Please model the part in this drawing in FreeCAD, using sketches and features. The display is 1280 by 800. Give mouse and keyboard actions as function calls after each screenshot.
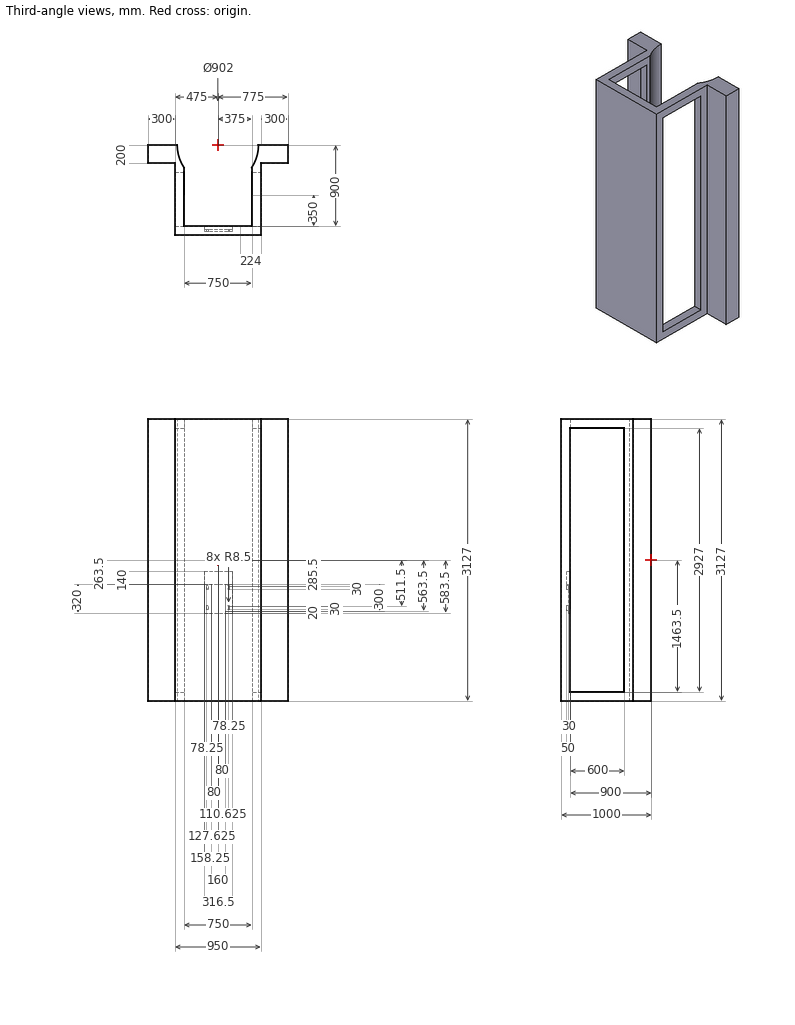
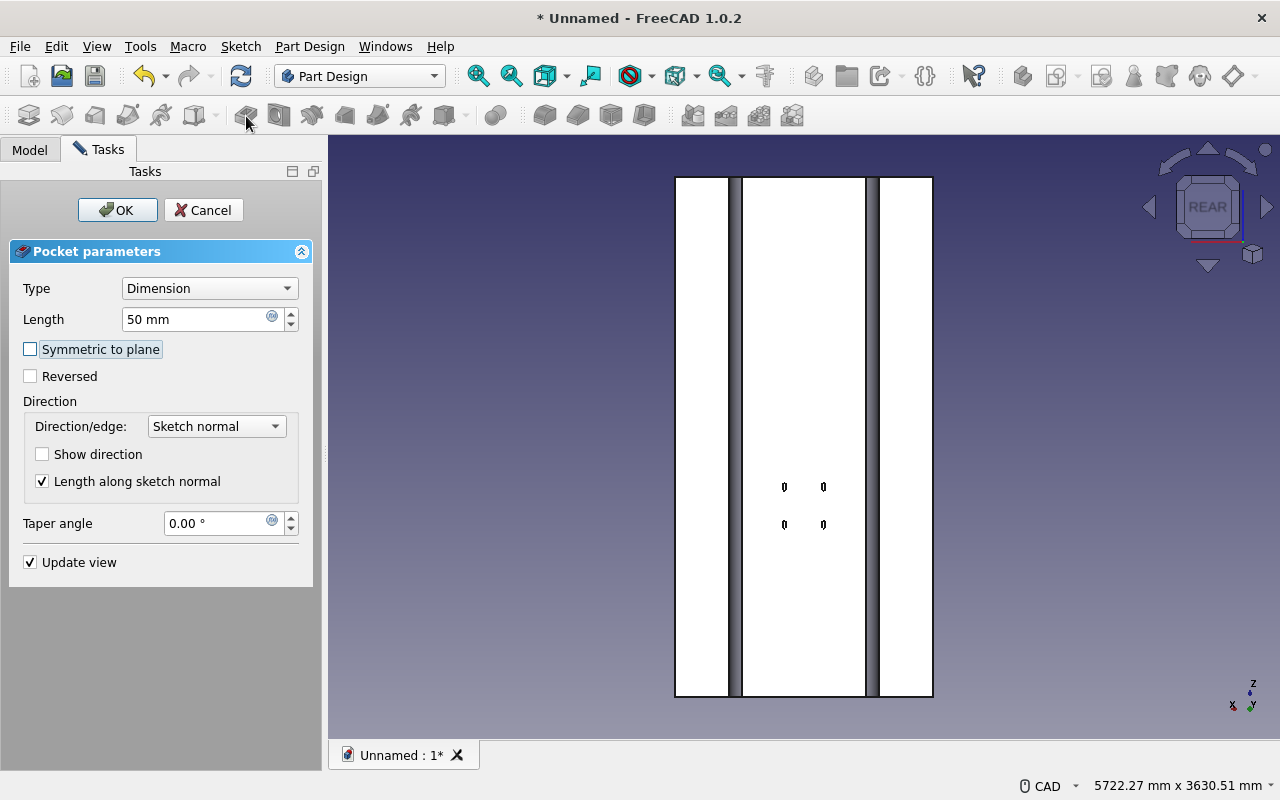
click(118, 210)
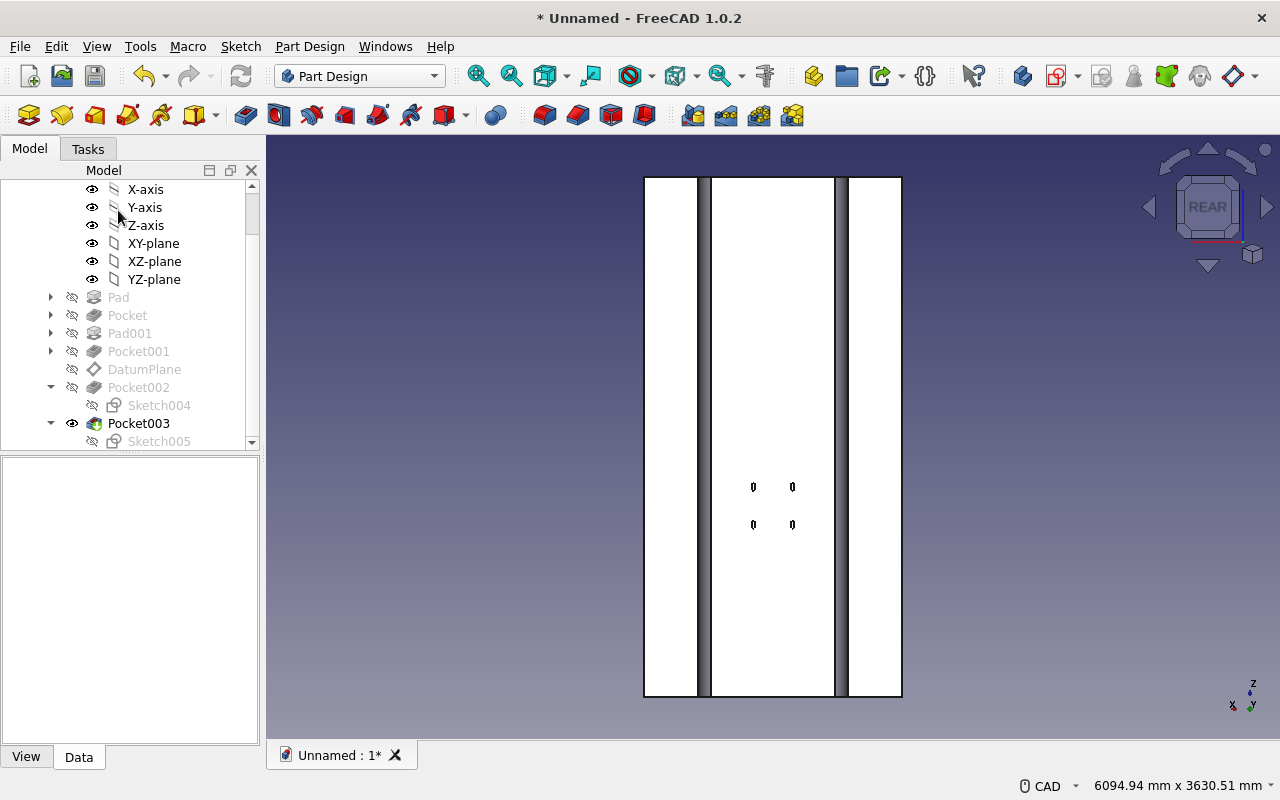
click(773, 287)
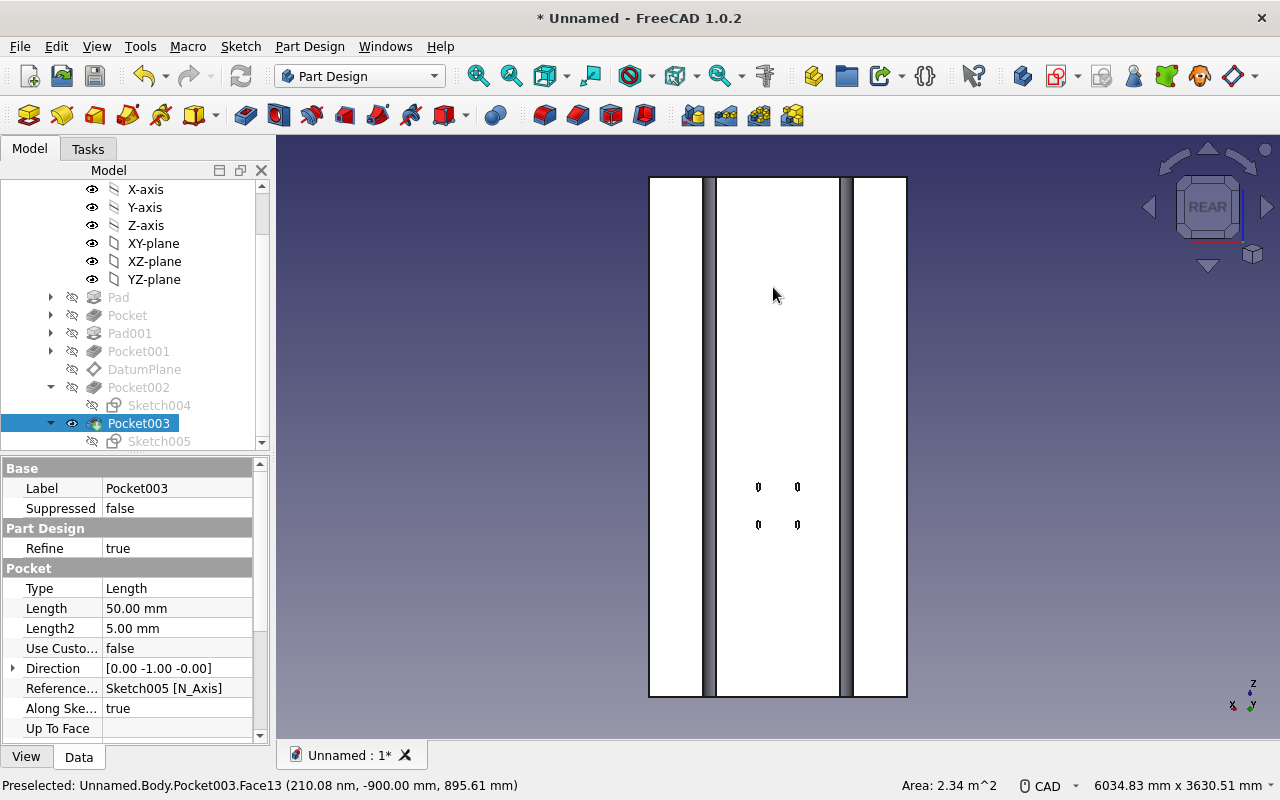
click(1056, 76)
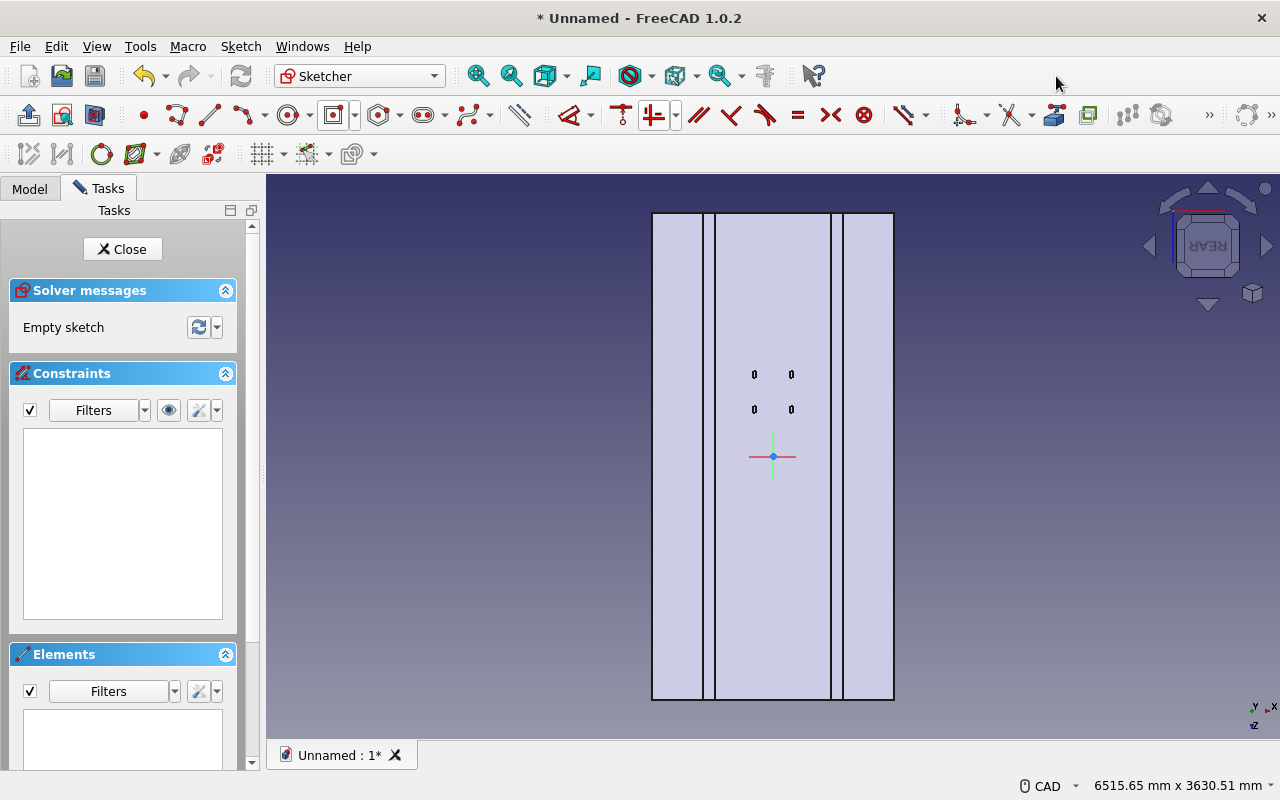
click(95, 116)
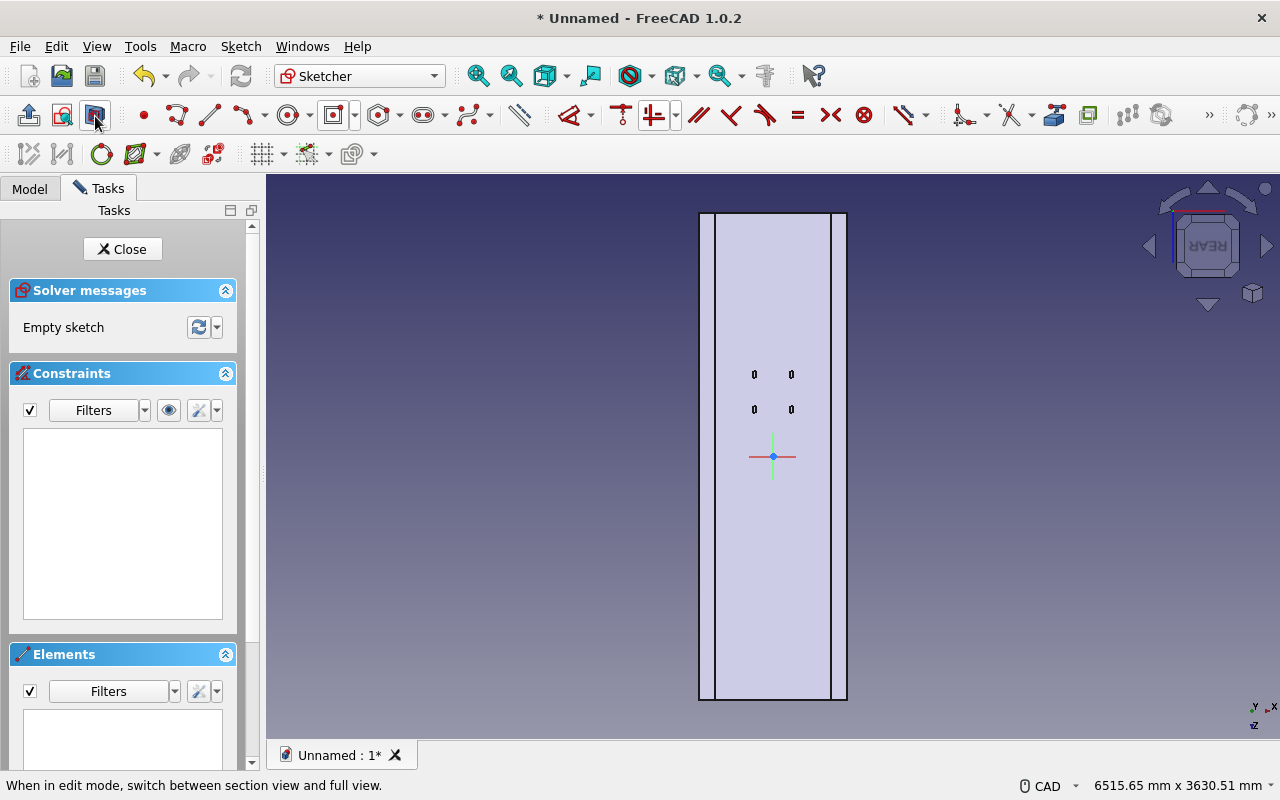
scroll(795, 398, up, 7)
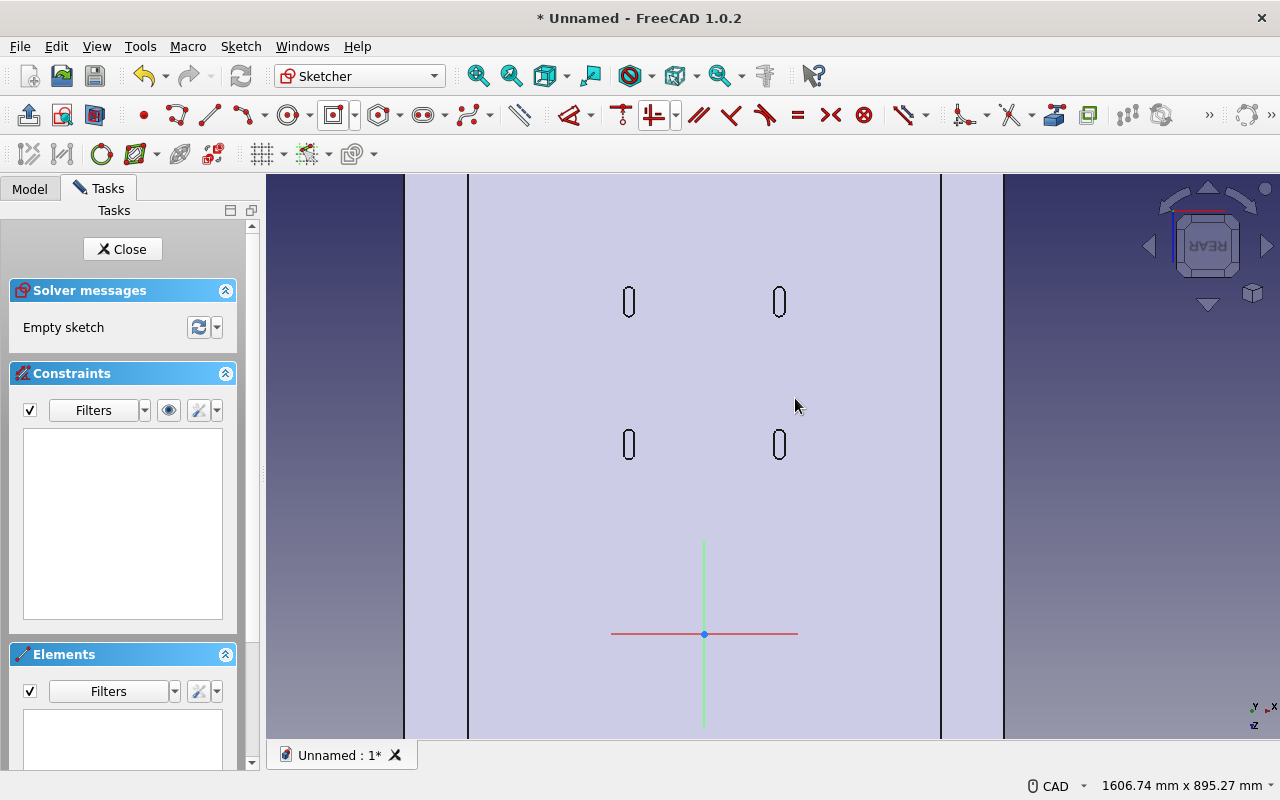
key(g)
key(r)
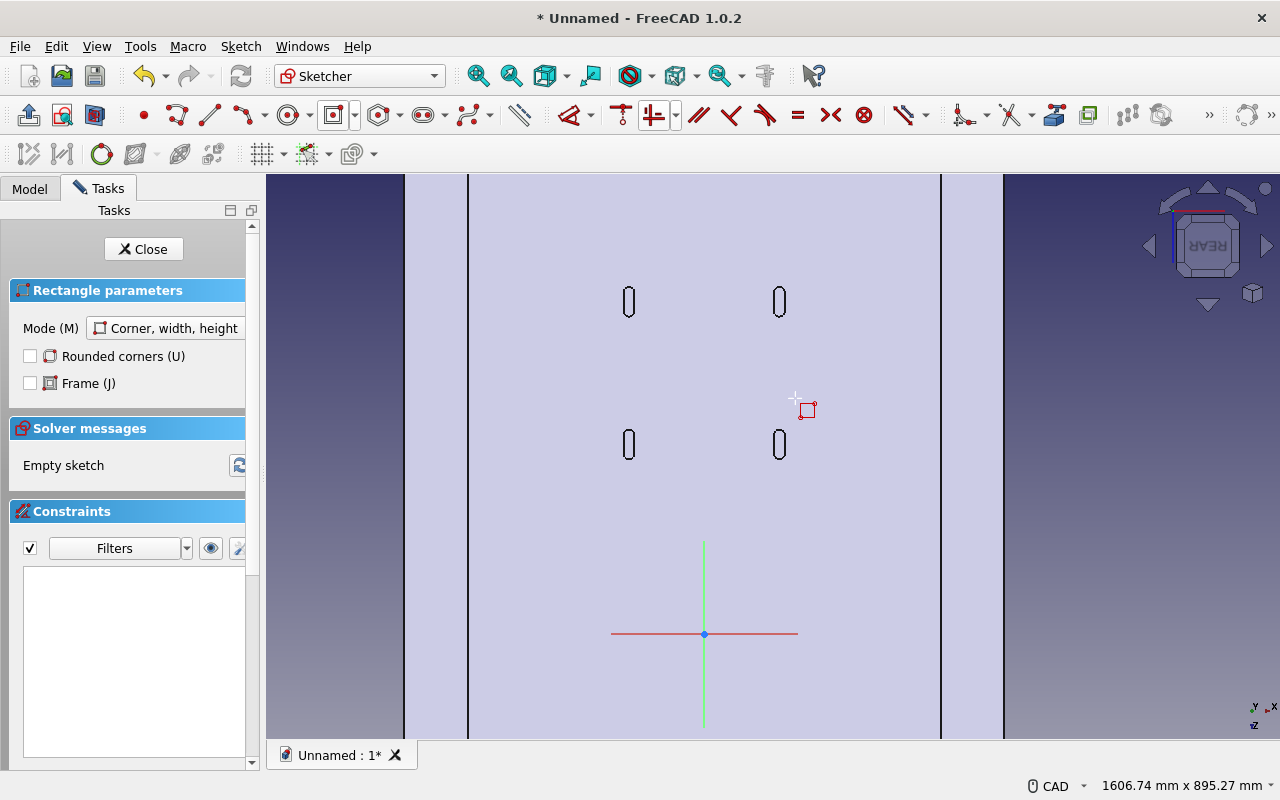
click(755, 278)
click(804, 468)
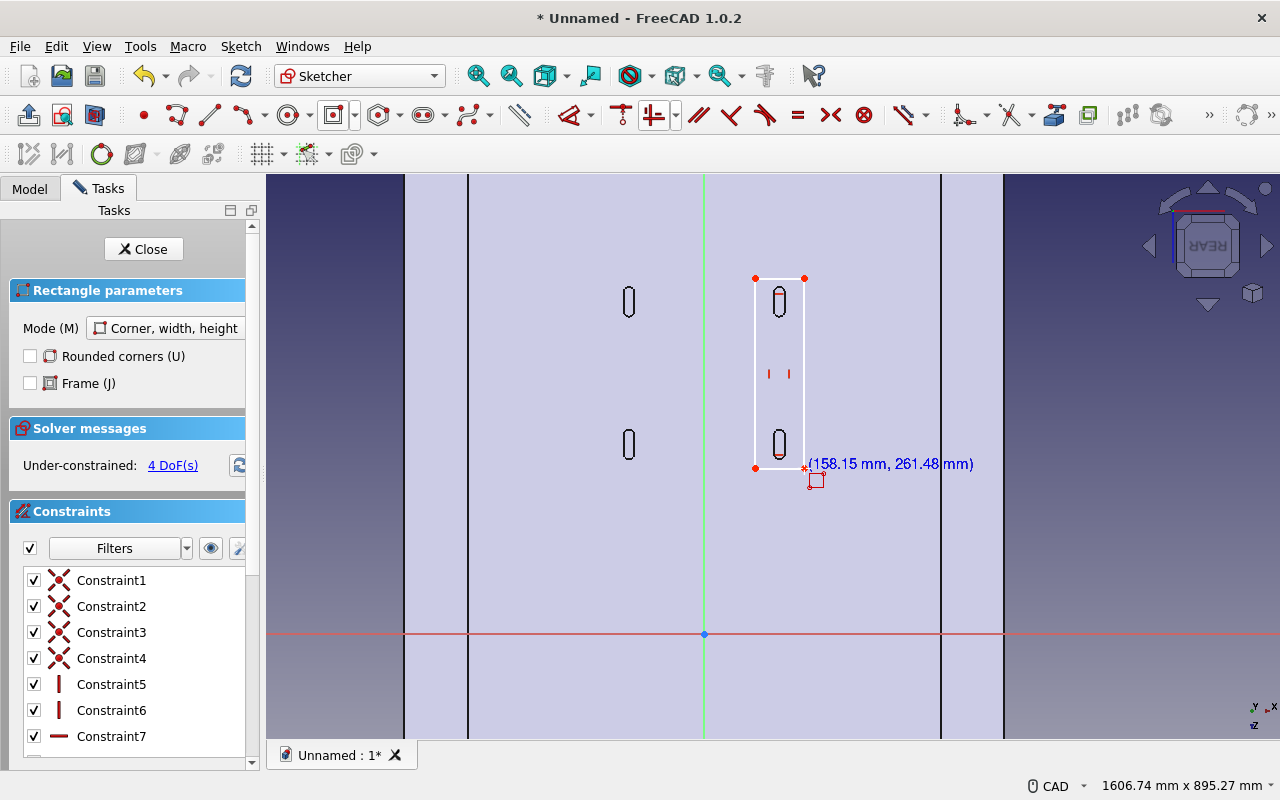
click(604, 278)
click(654, 468)
key(Escape)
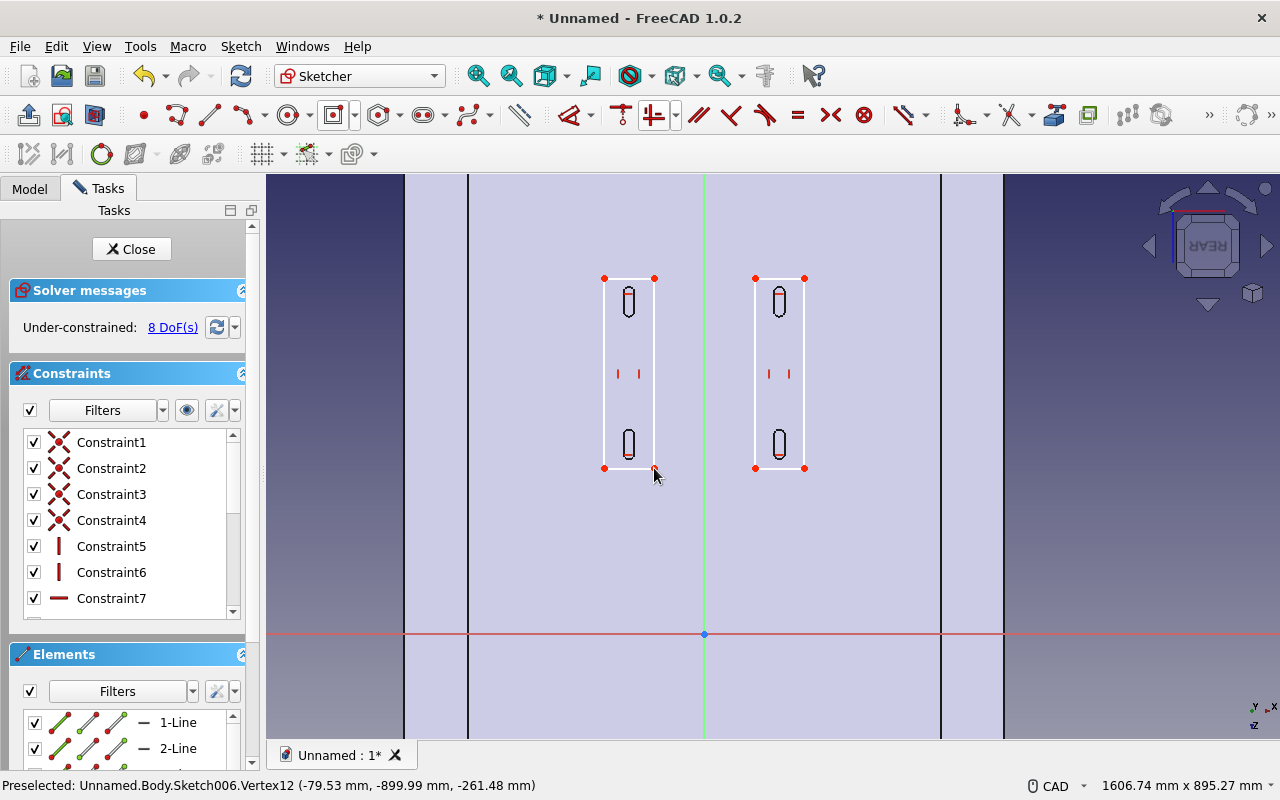
click(568, 116)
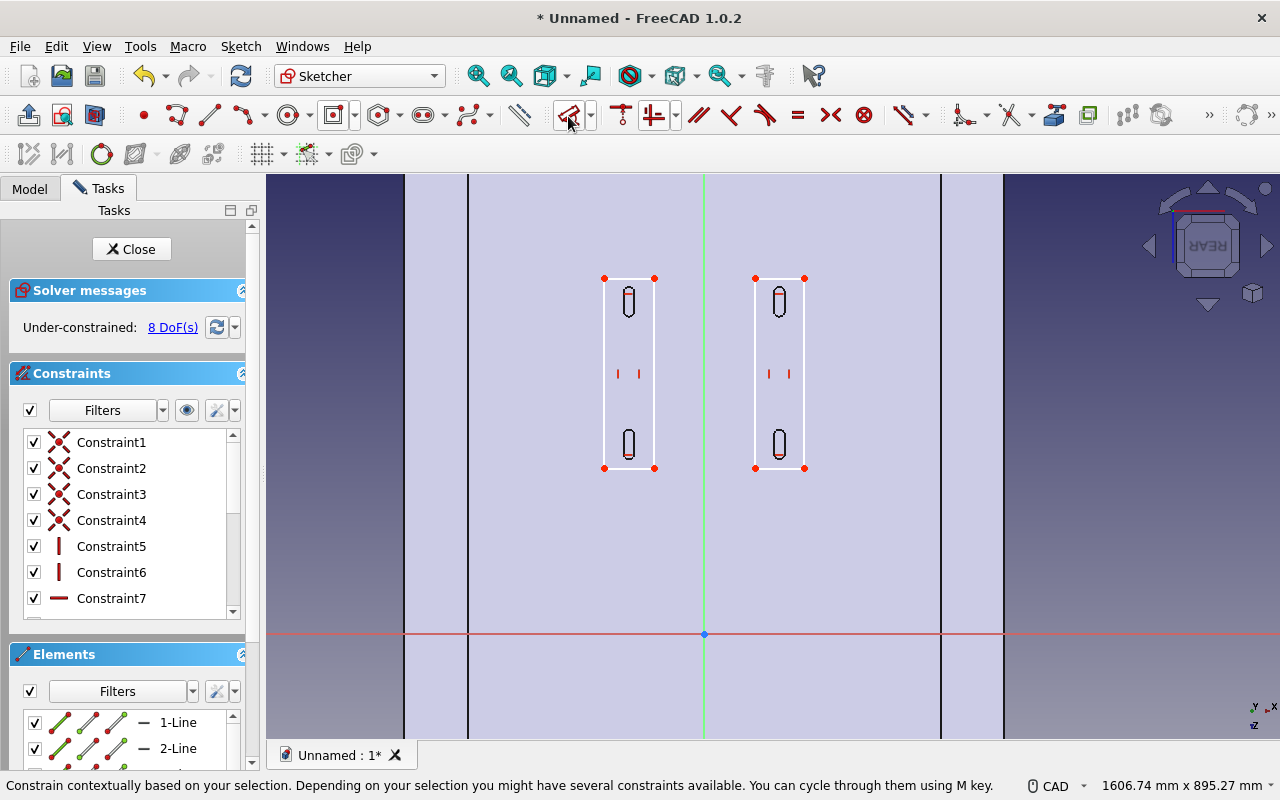
click(755, 336)
click(789, 374)